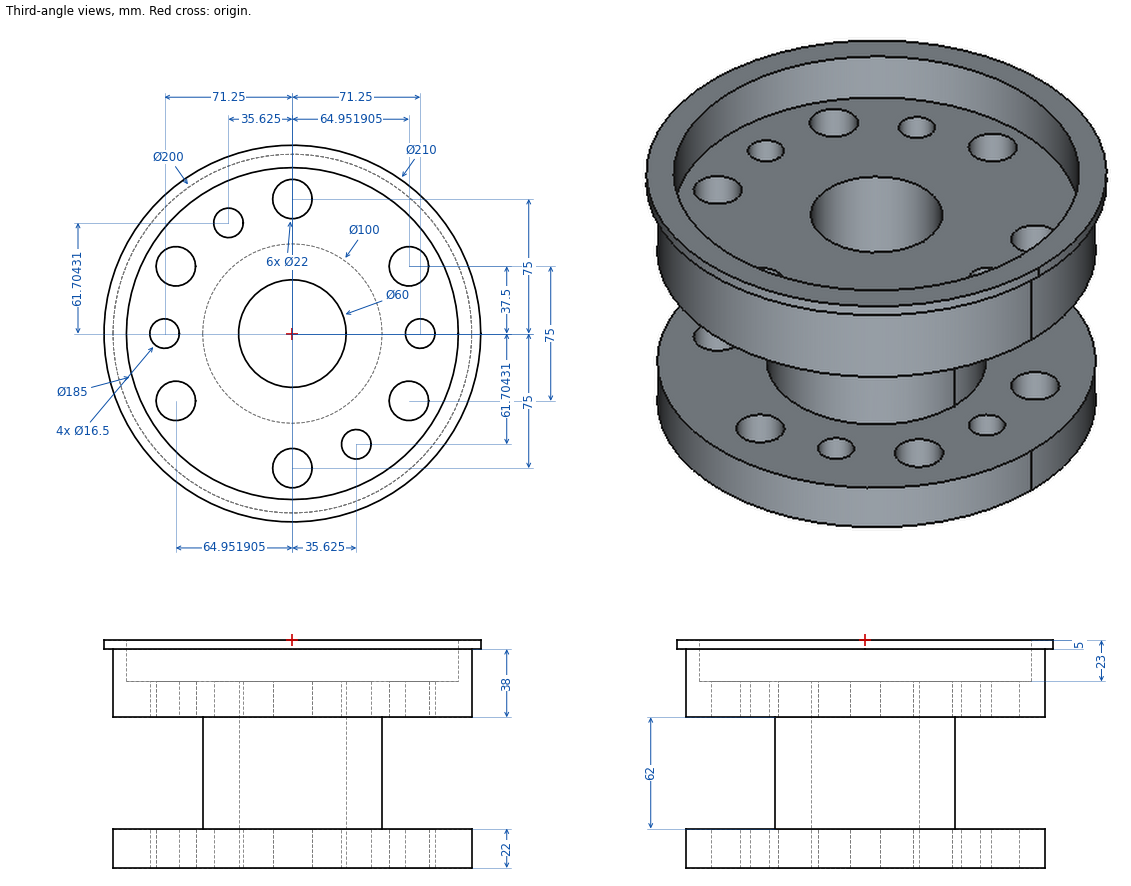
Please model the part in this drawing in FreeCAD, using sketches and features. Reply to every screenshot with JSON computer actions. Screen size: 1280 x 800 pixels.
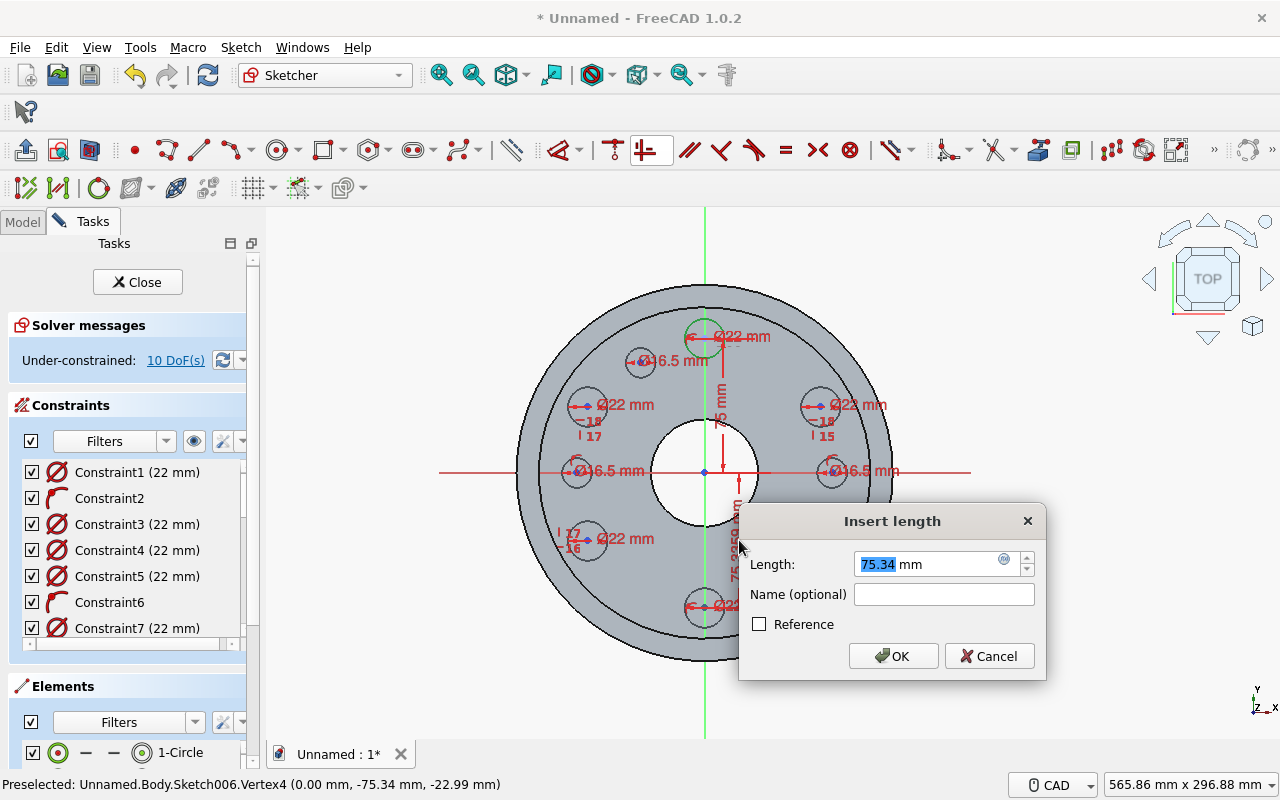
{"action": "type", "text": "75"}
{"action": "key", "text": "Return"}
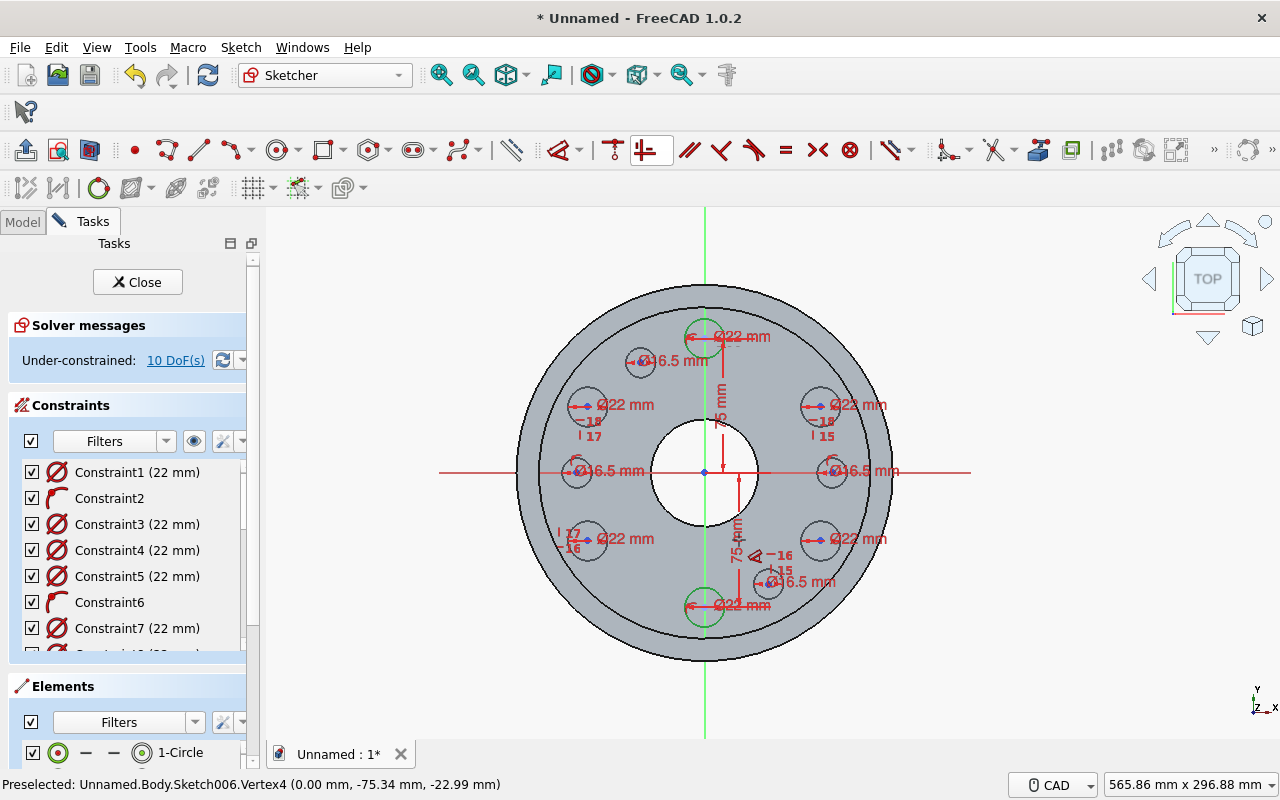
{"action": "left_click", "coordinate": [821, 407]}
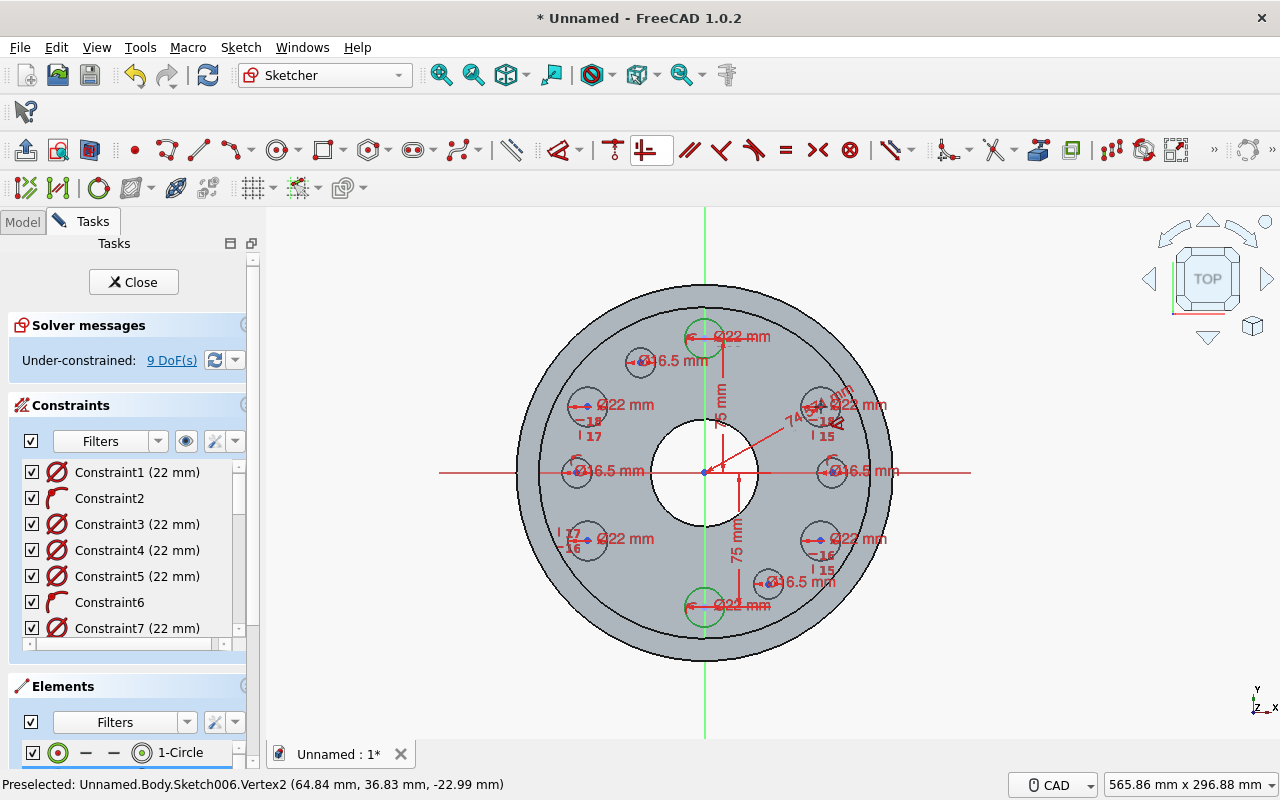
{"action": "left_click", "coordinate": [821, 541]}
{"action": "left_click", "coordinate": [855, 443]}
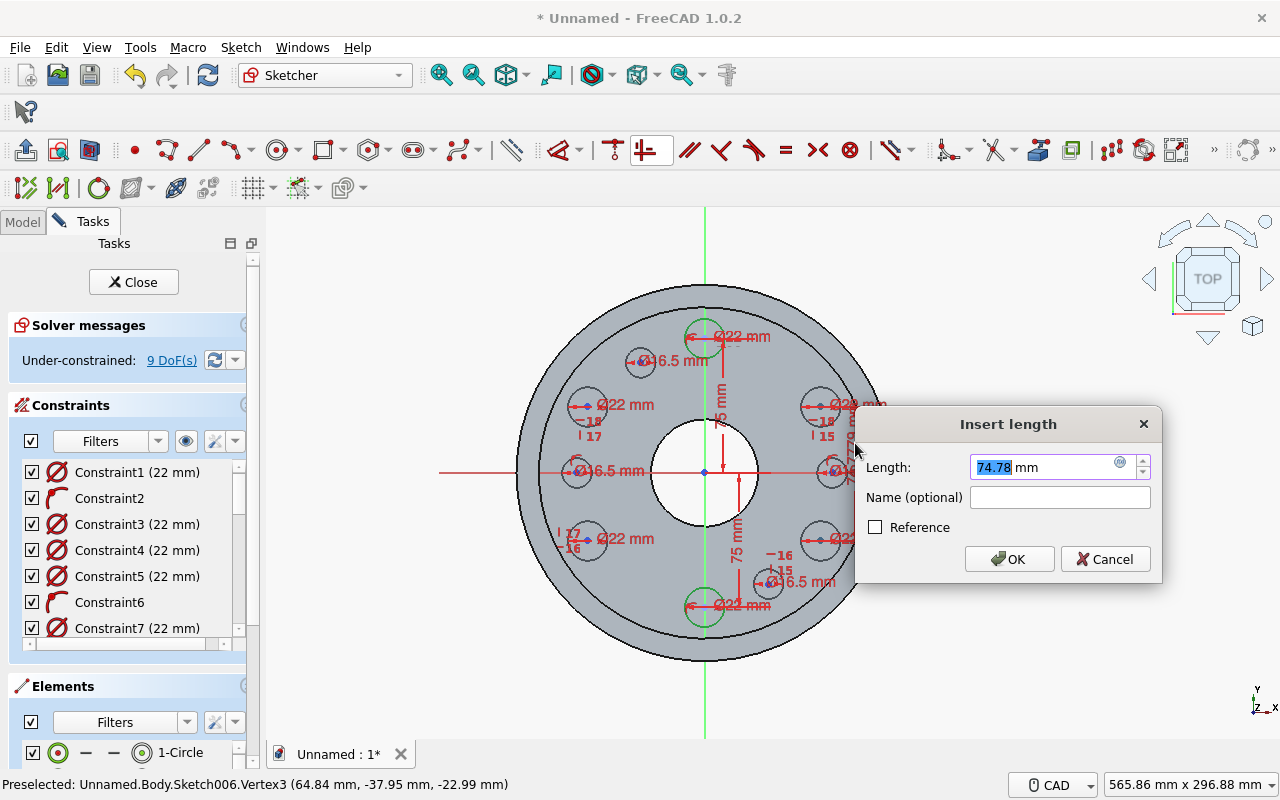
{"action": "type", "text": "75"}
{"action": "key", "text": "Return"}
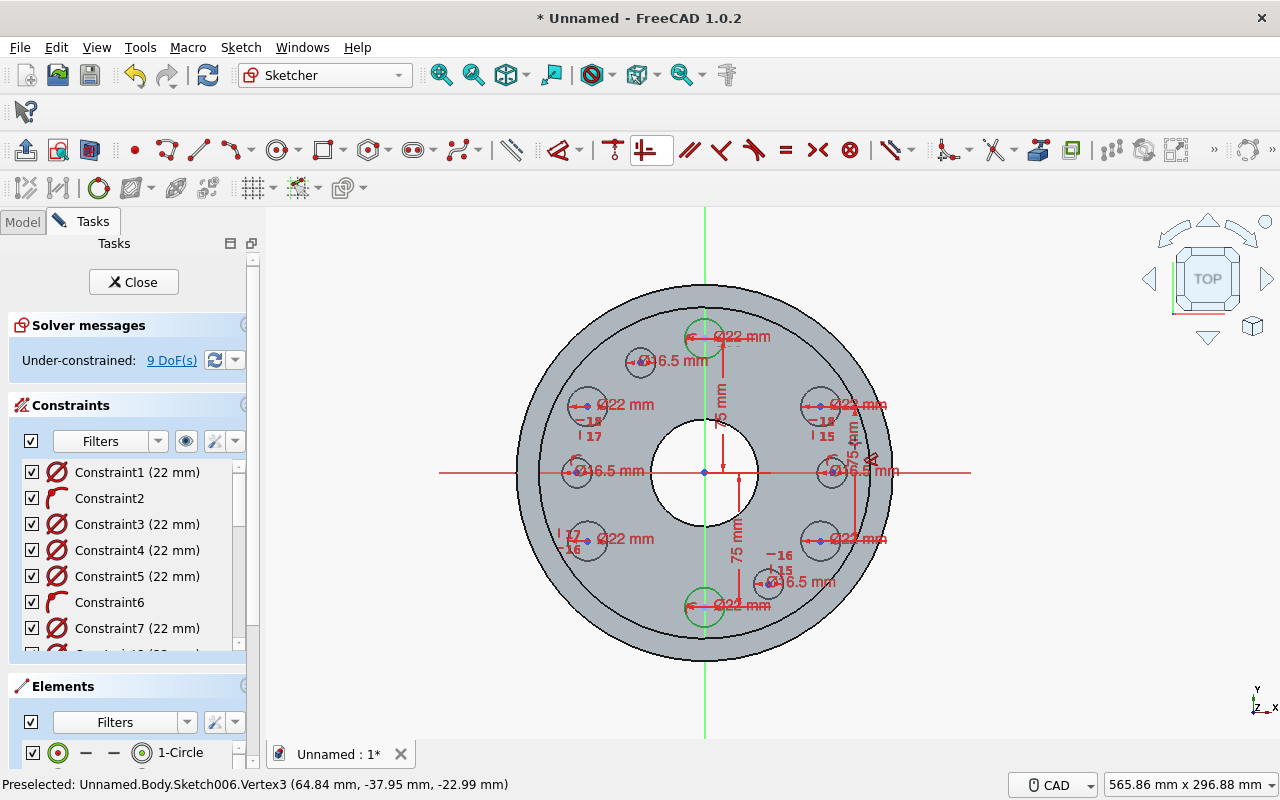
{"action": "left_click", "coordinate": [821, 407]}
{"action": "left_click", "coordinate": [855, 417]}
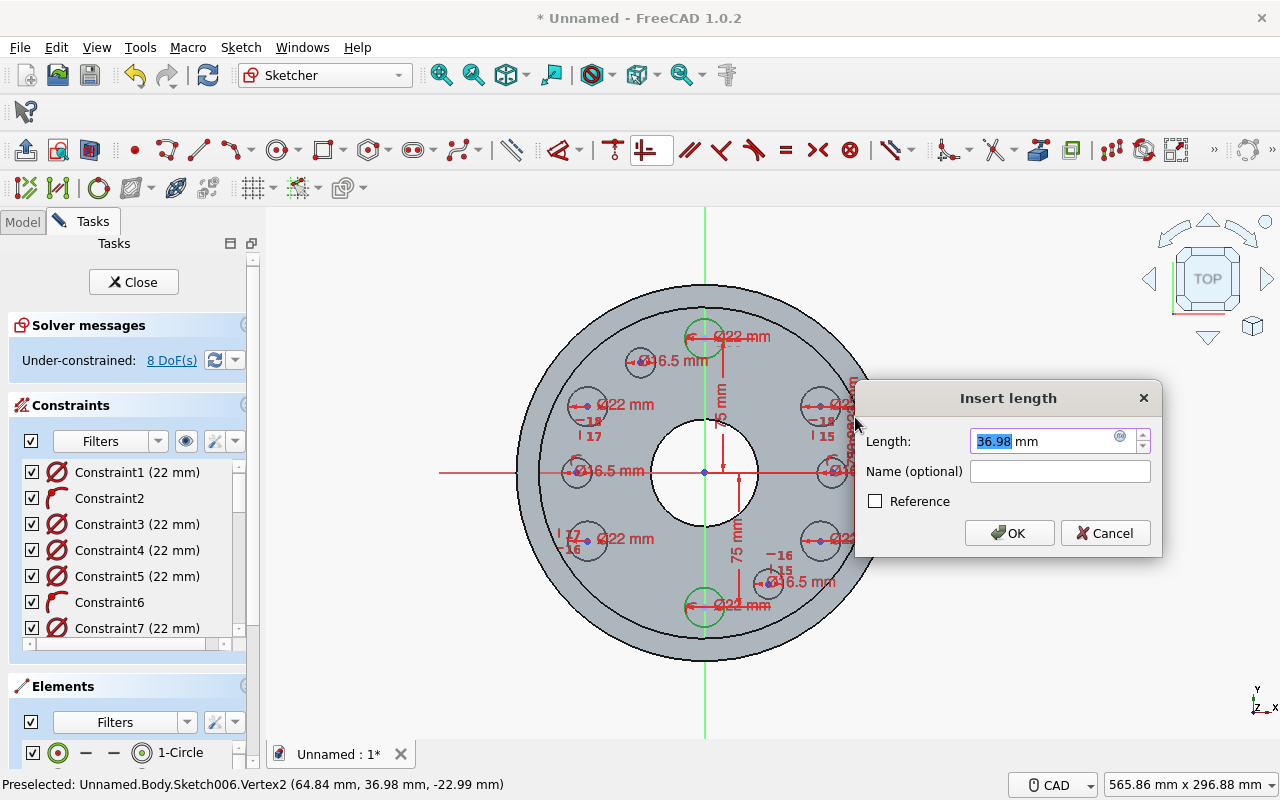
{"action": "type", "text": "37.5"}
{"action": "key", "text": "Return"}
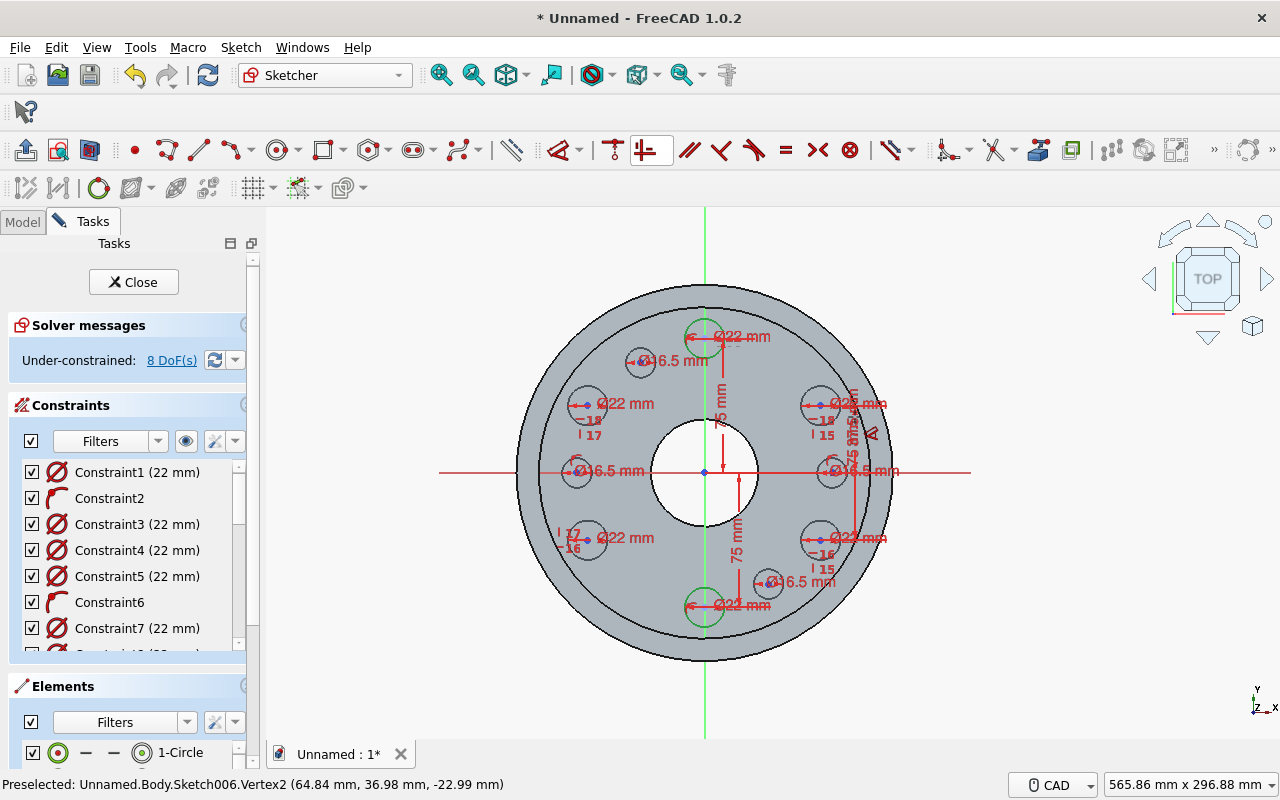
{"action": "left_click", "coordinate": [577, 473]}
{"action": "left_click", "coordinate": [641, 507]}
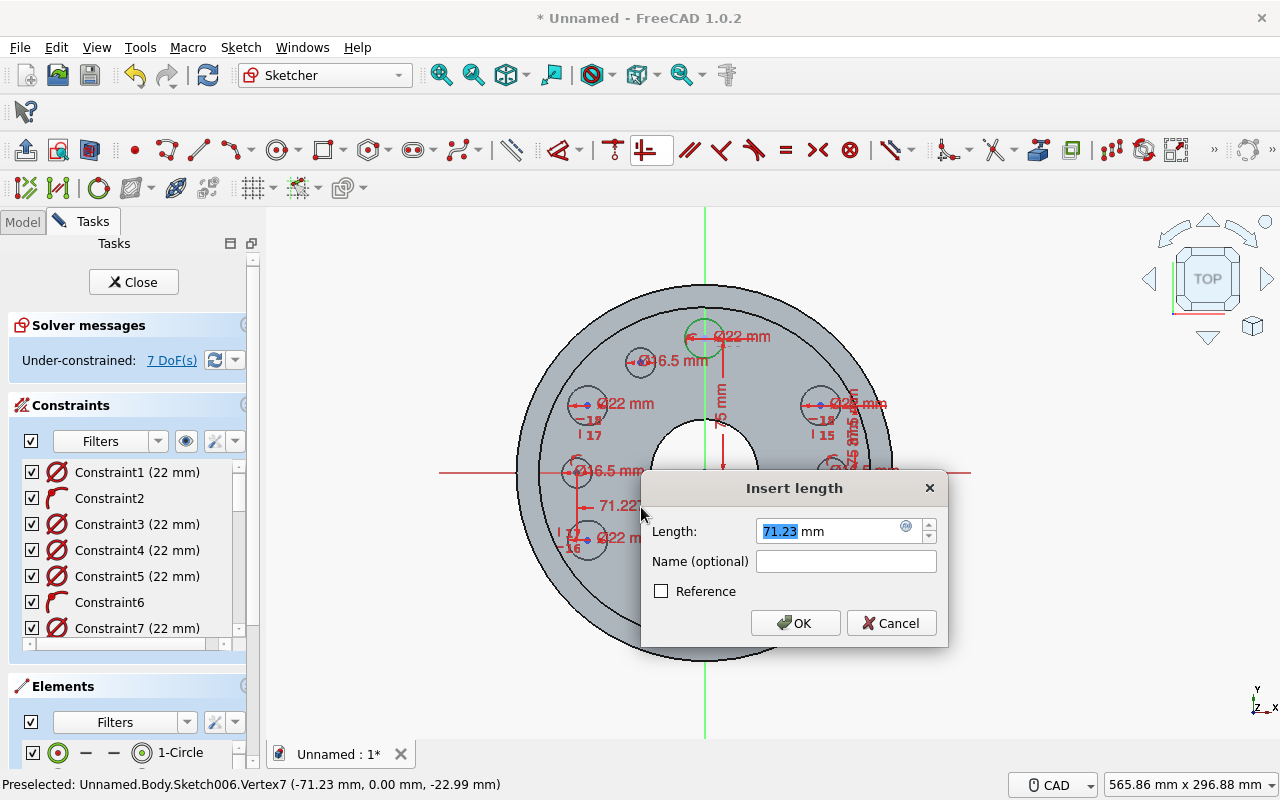
{"action": "type", "text": "71.25"}
{"action": "key", "text": "Return"}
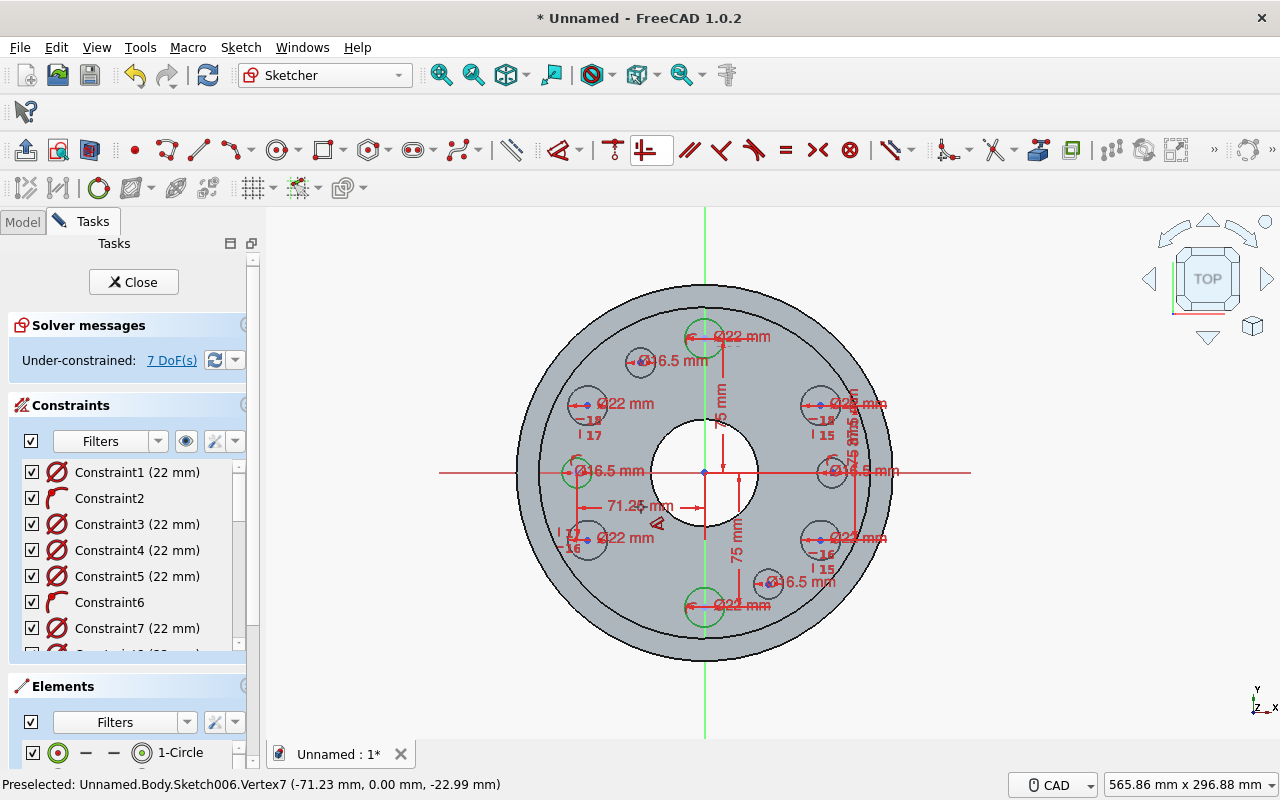
{"action": "left_click", "coordinate": [832, 473]}
{"action": "left_click", "coordinate": [768, 507]}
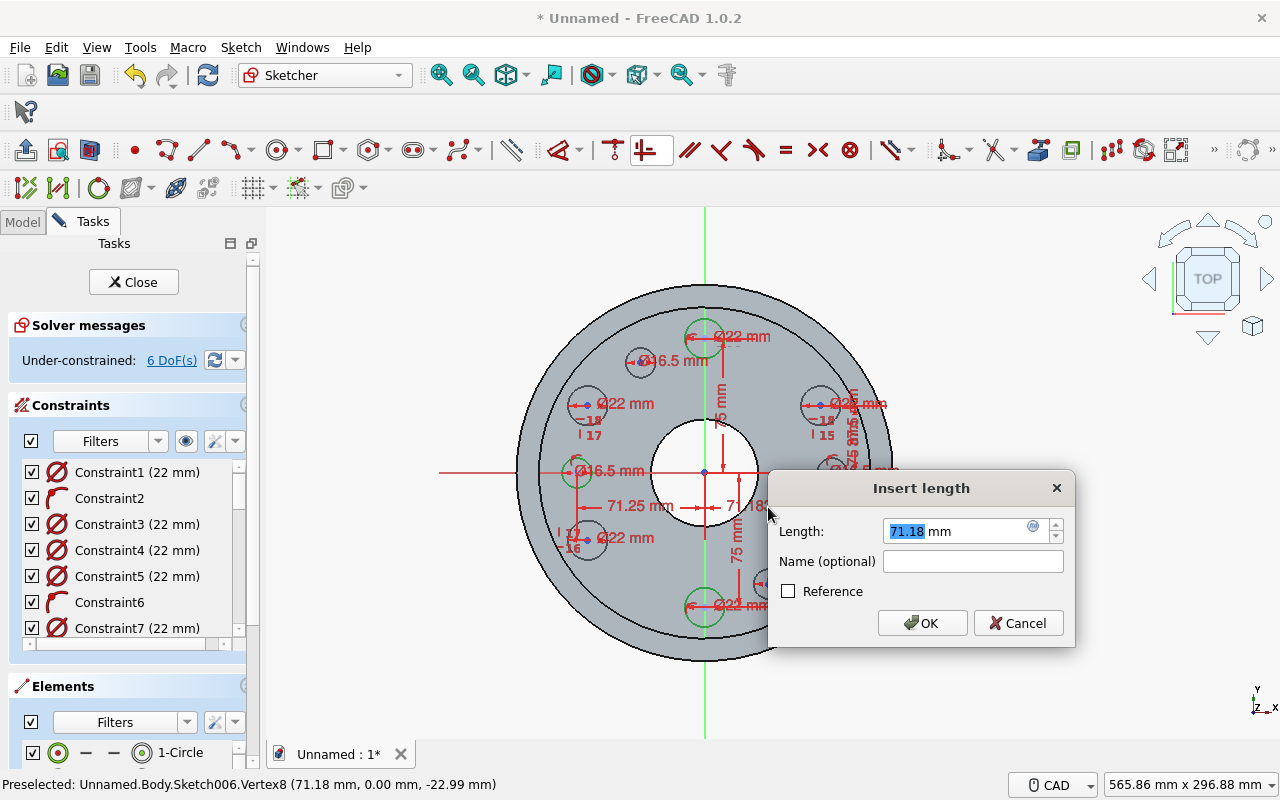
{"action": "type", "text": "71.25"}
{"action": "key", "text": "Return"}